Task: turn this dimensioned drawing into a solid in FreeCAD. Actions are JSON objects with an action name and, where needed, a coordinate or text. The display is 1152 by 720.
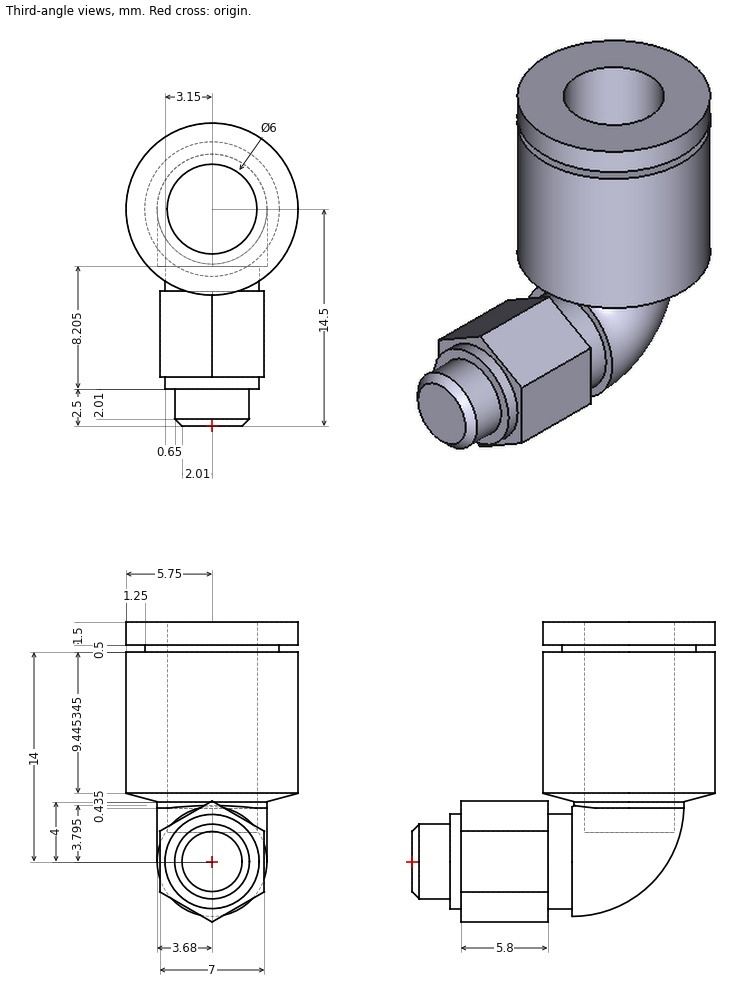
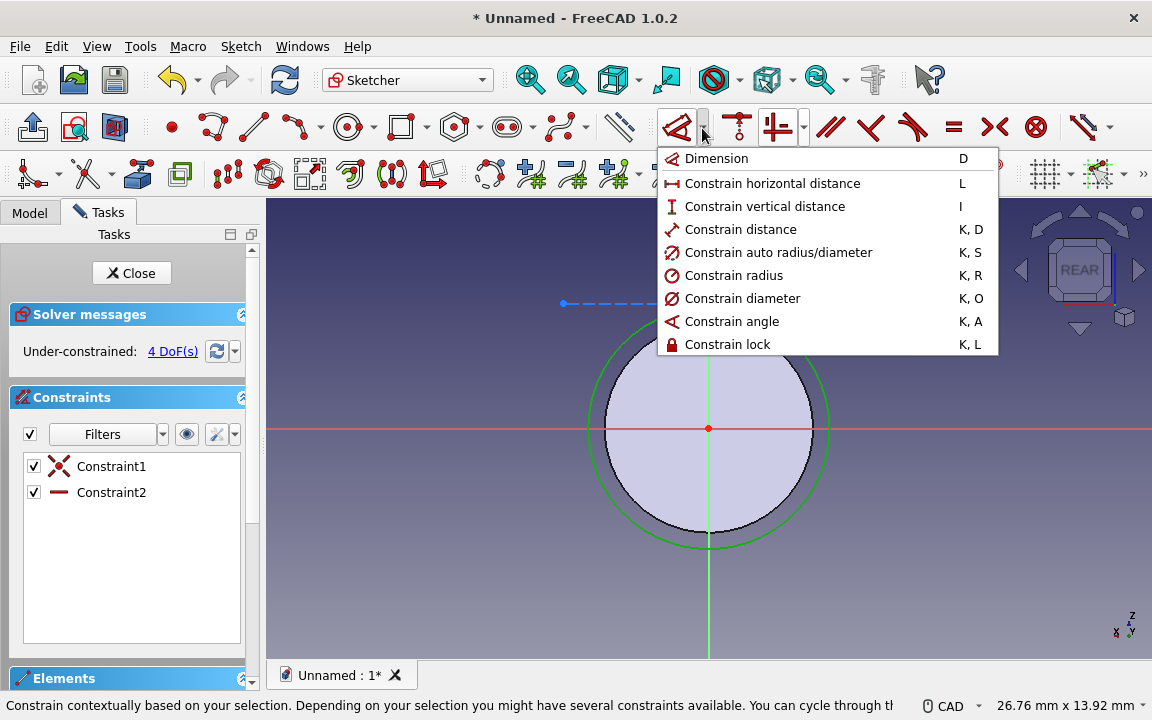
{"action": "left_click", "coordinate": [828, 298]}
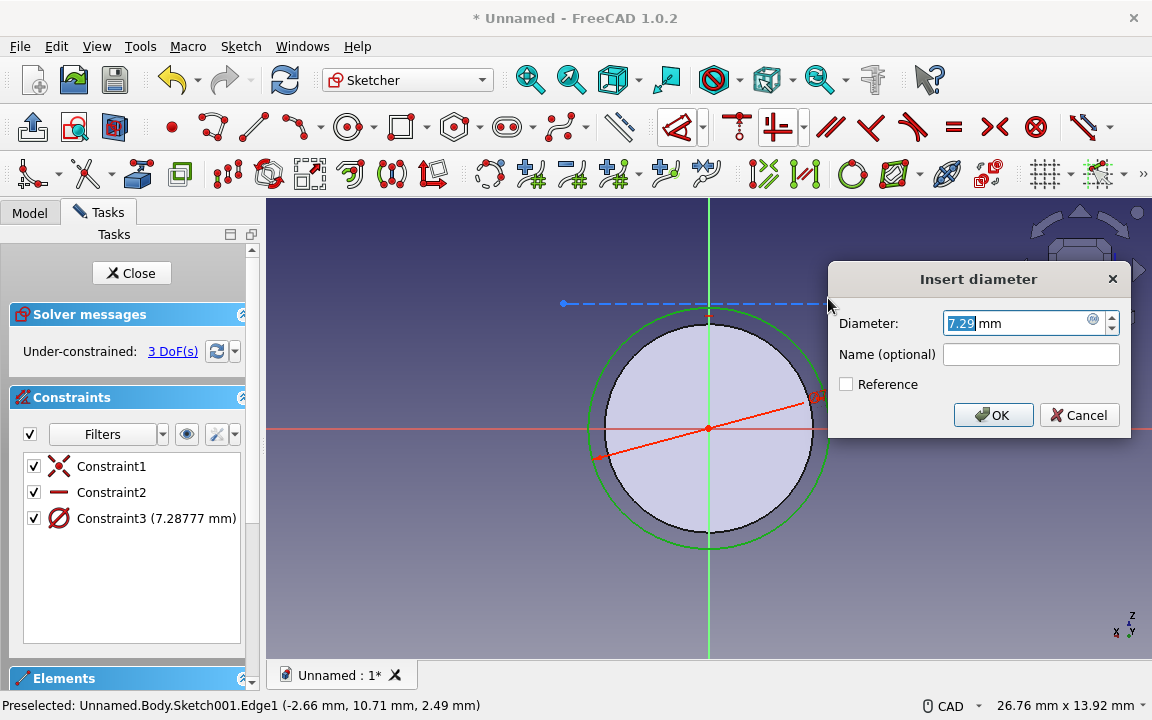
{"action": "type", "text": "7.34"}
{"action": "key", "text": "Return"}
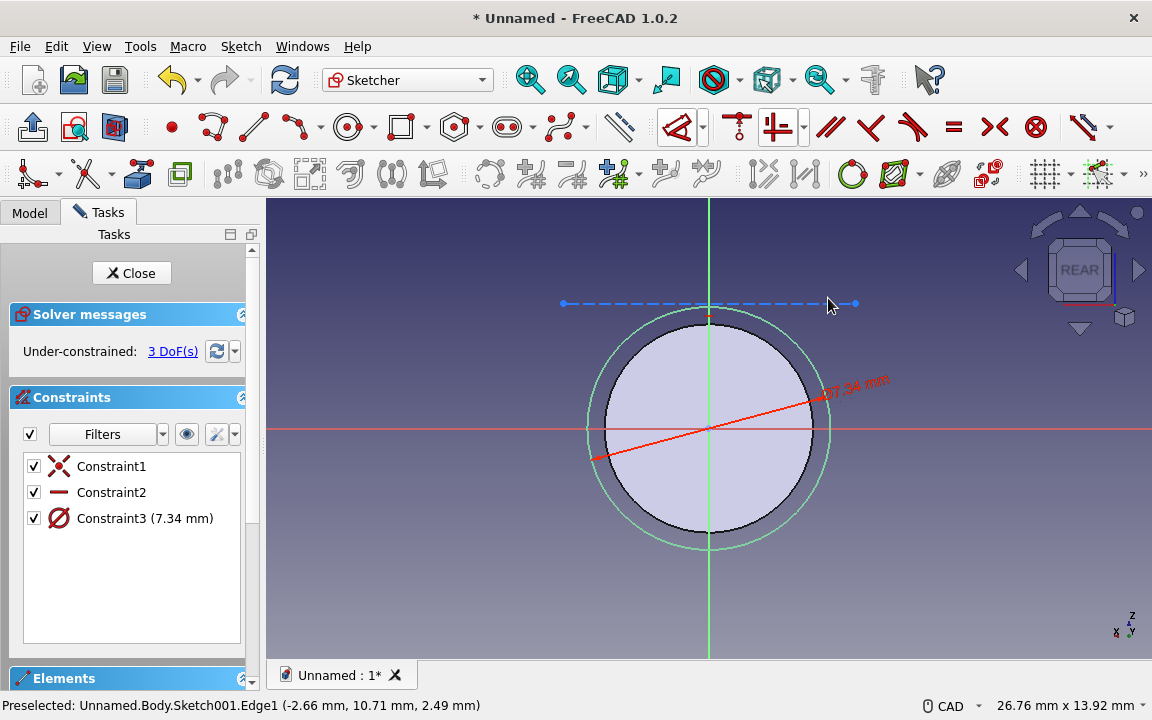
{"action": "scroll", "coordinate": [855, 304], "scroll_direction": "up", "scroll_amount": 4}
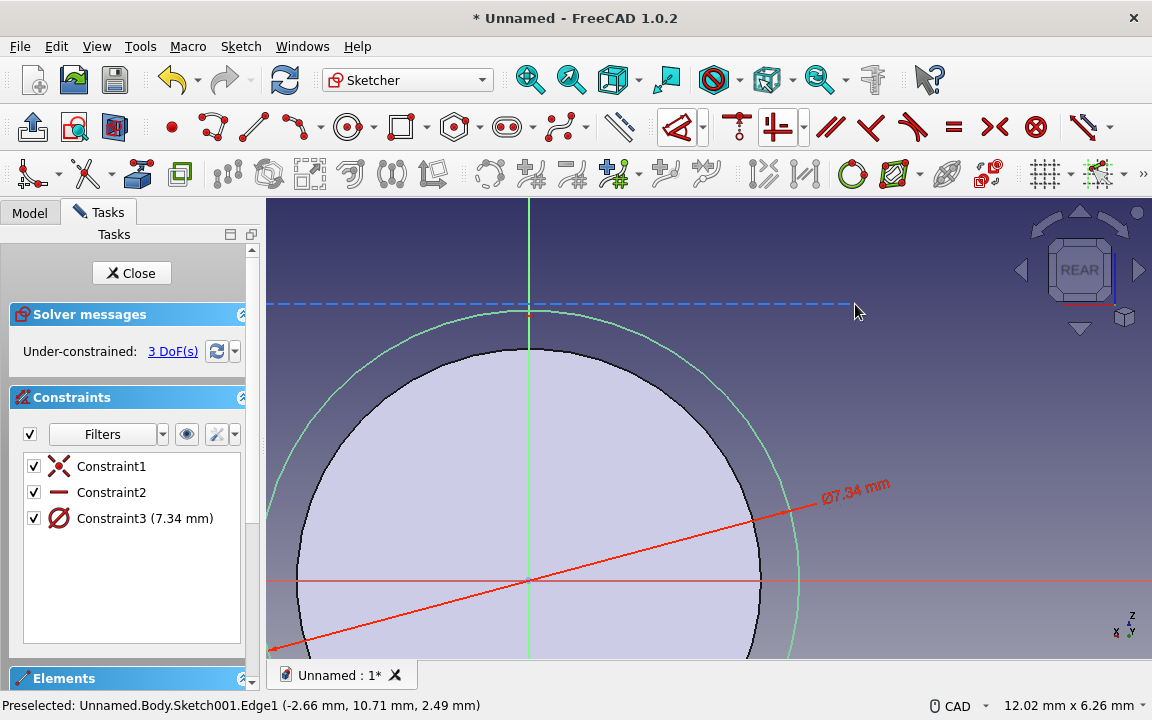
{"action": "left_click", "coordinate": [854, 304]}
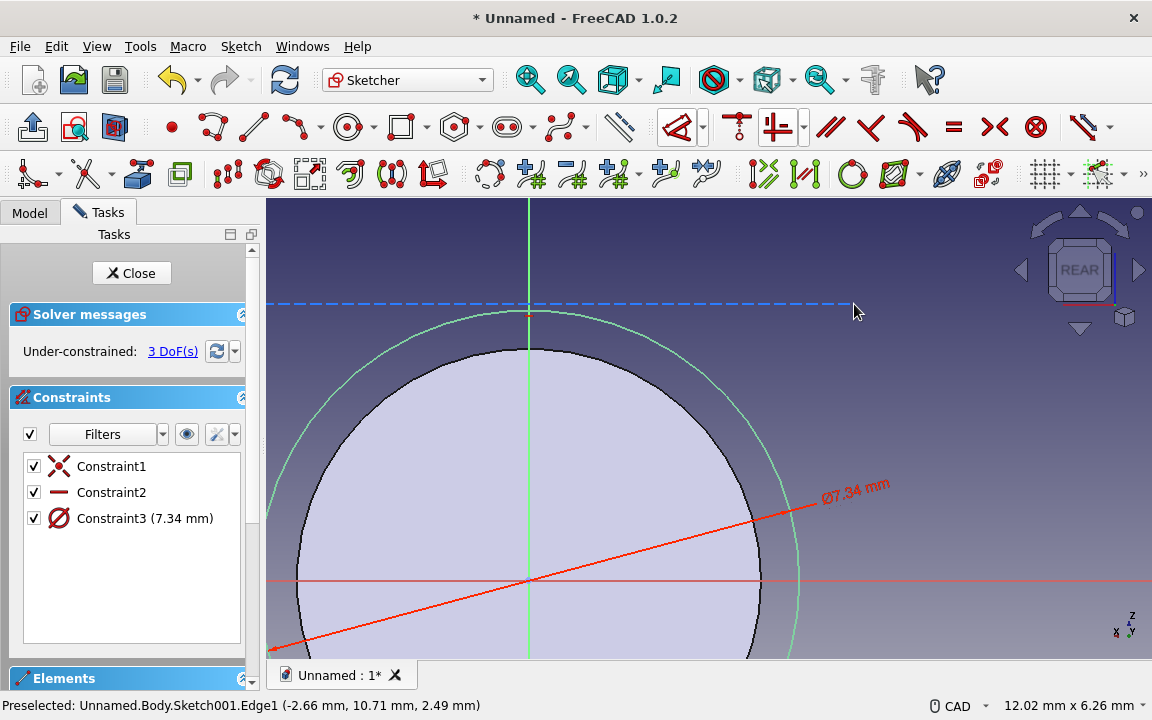
{"action": "key", "text": "i"}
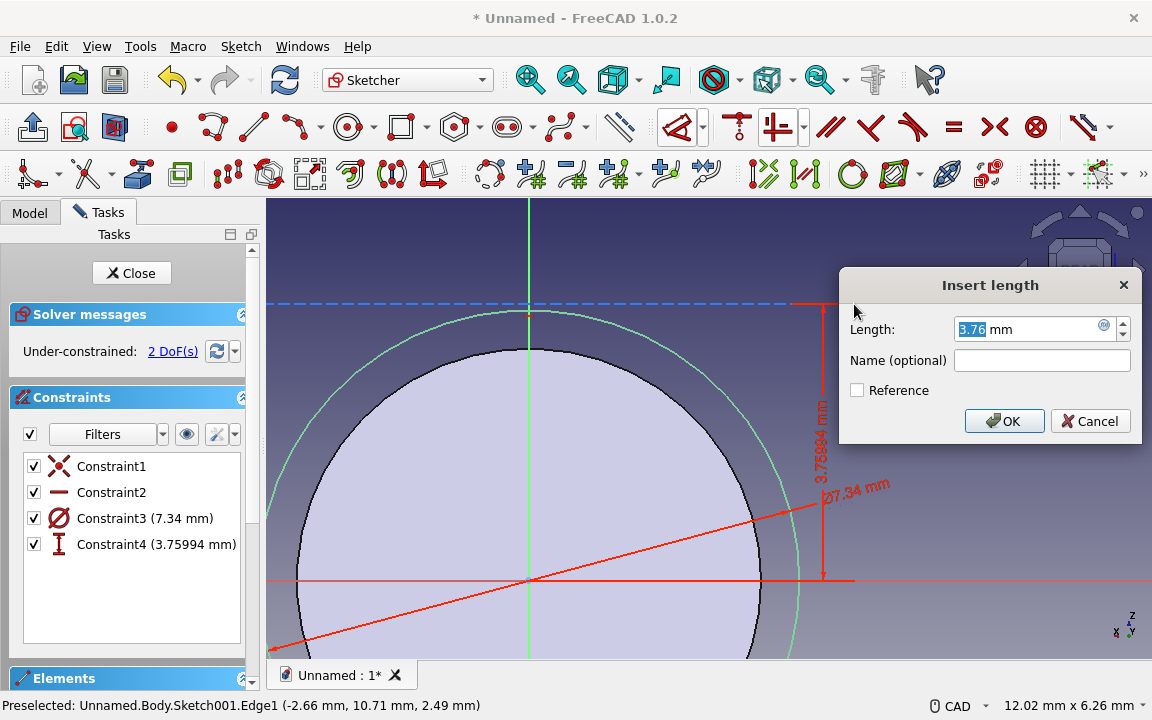
{"action": "type", "text": "3.795"}
{"action": "key", "text": "Return"}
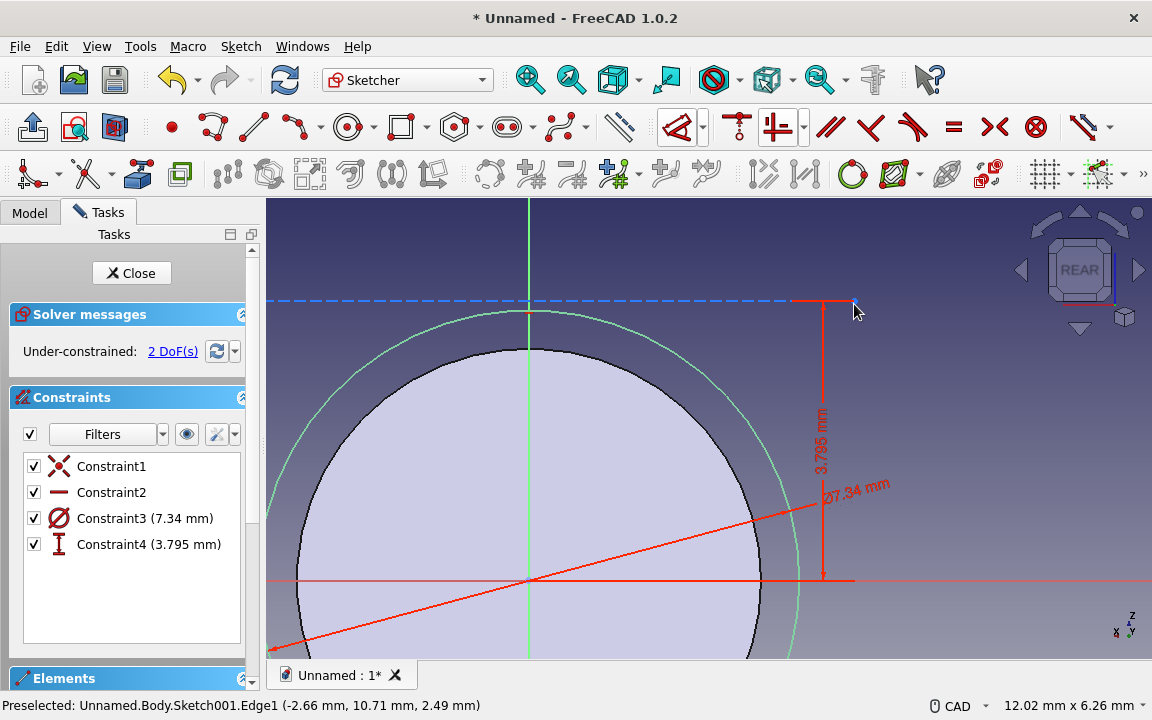
{"action": "left_click", "coordinate": [132, 273]}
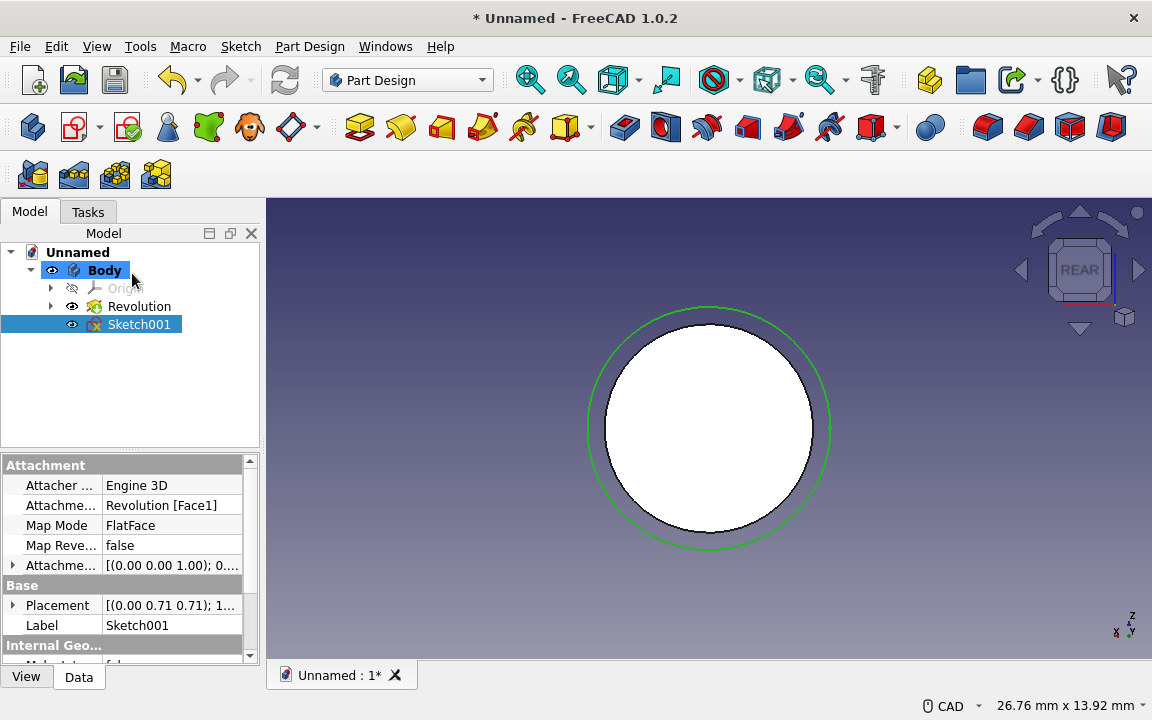
{"action": "left_click", "coordinate": [401, 128]}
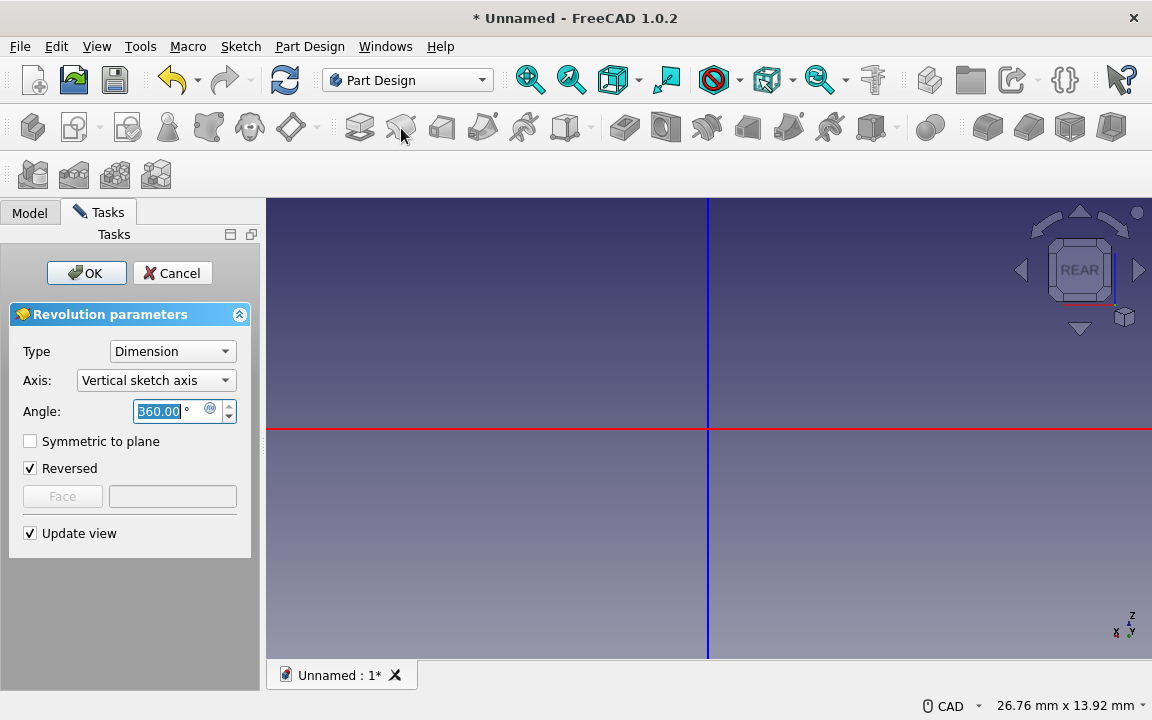
{"action": "left_click", "coordinate": [157, 380]}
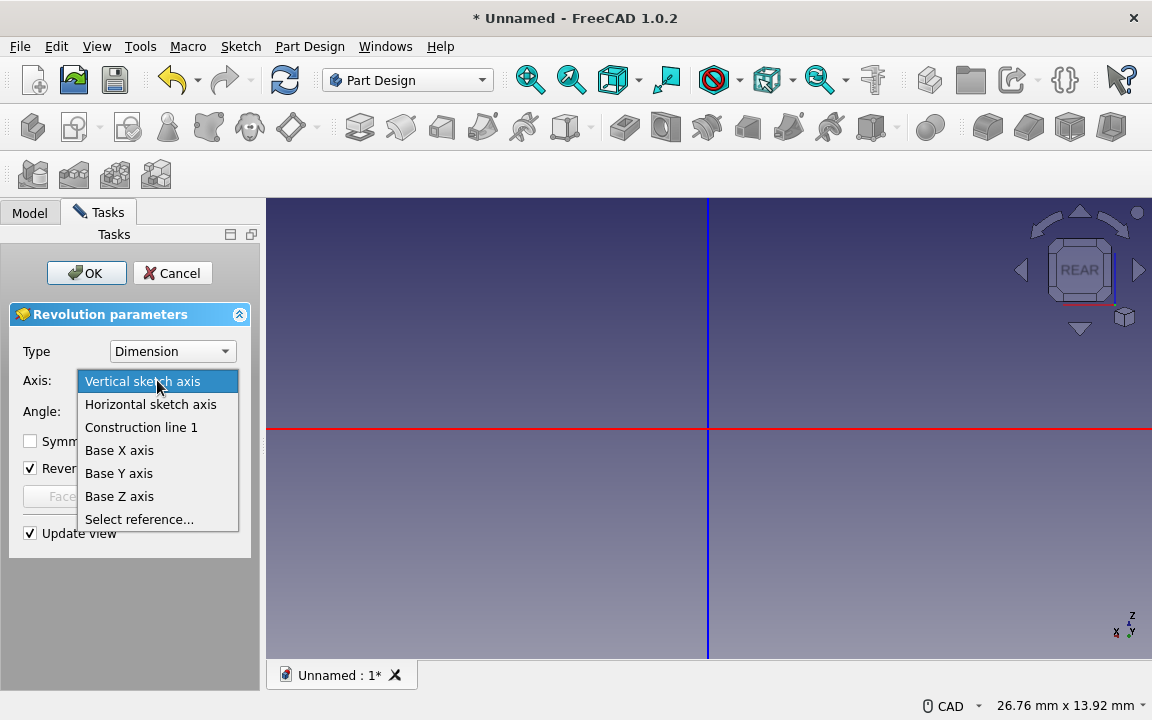
{"action": "left_click", "coordinate": [156, 428]}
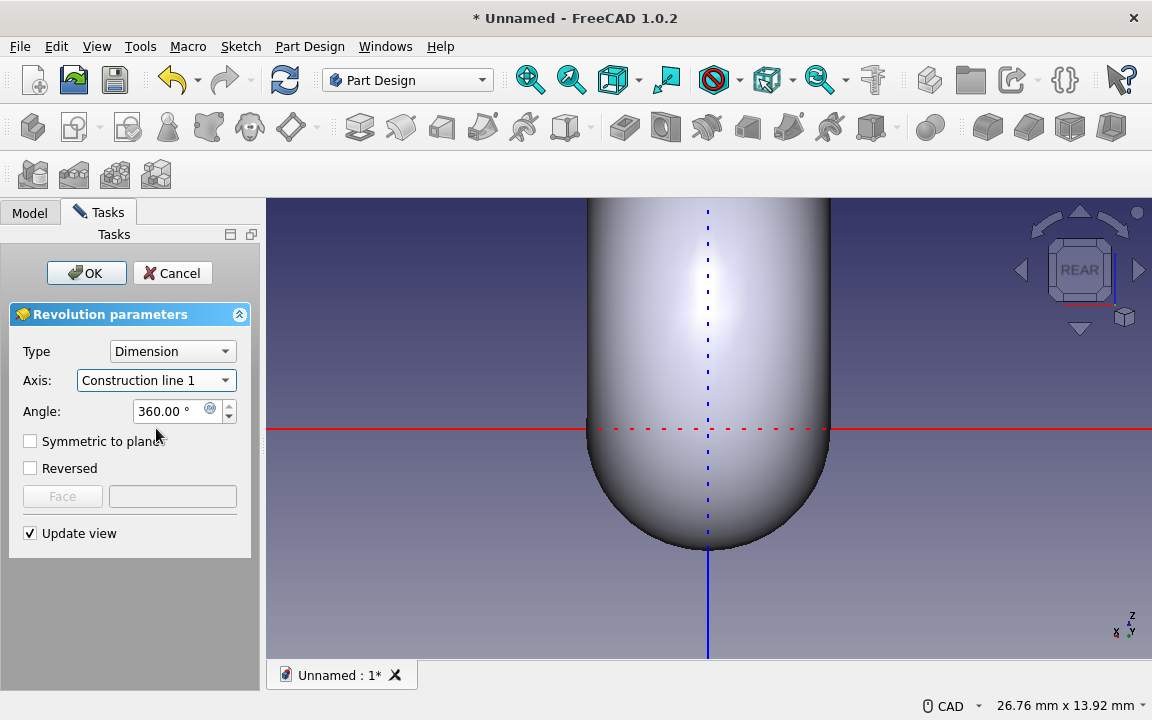
{"action": "triple_click", "coordinate": [178, 412]}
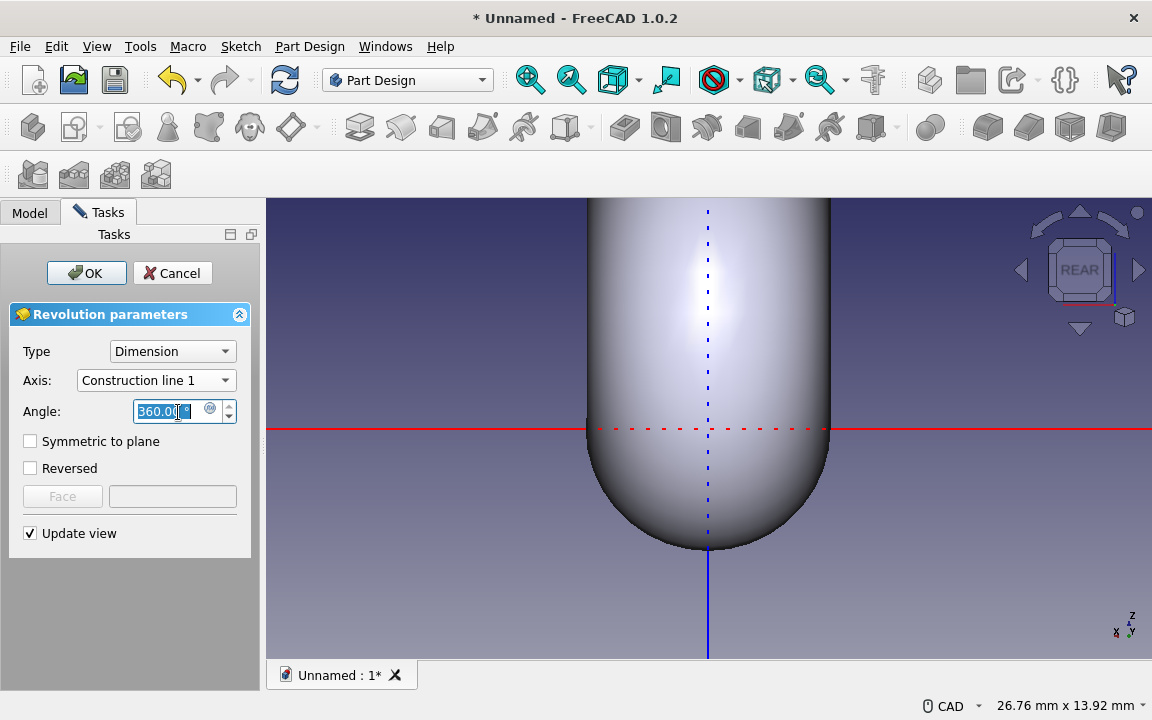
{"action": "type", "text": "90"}
{"action": "key", "text": "Tab"}